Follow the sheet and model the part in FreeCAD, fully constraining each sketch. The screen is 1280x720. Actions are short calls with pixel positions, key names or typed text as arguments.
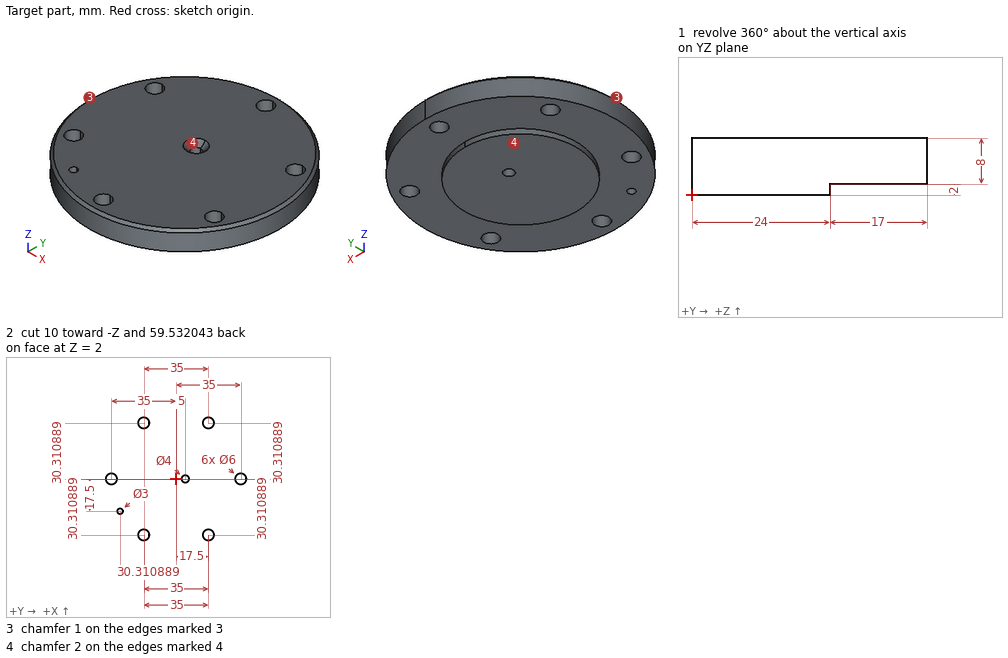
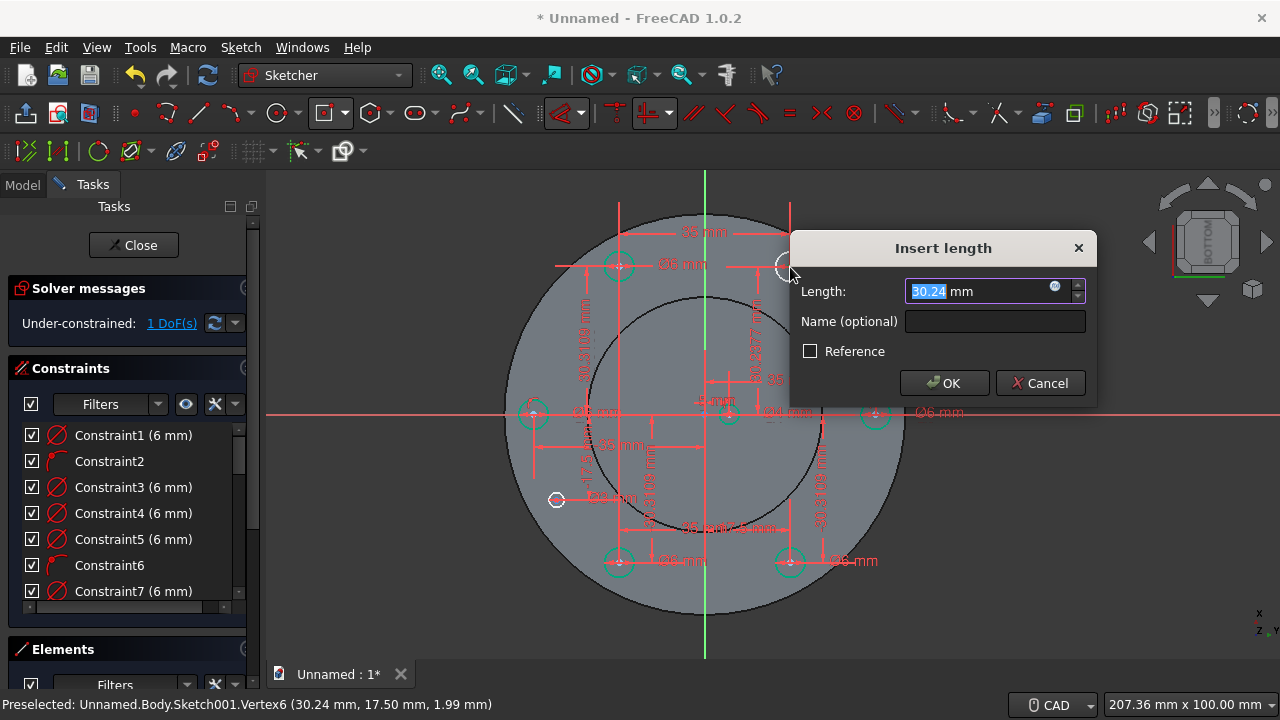
text(30.310889)
key(Return)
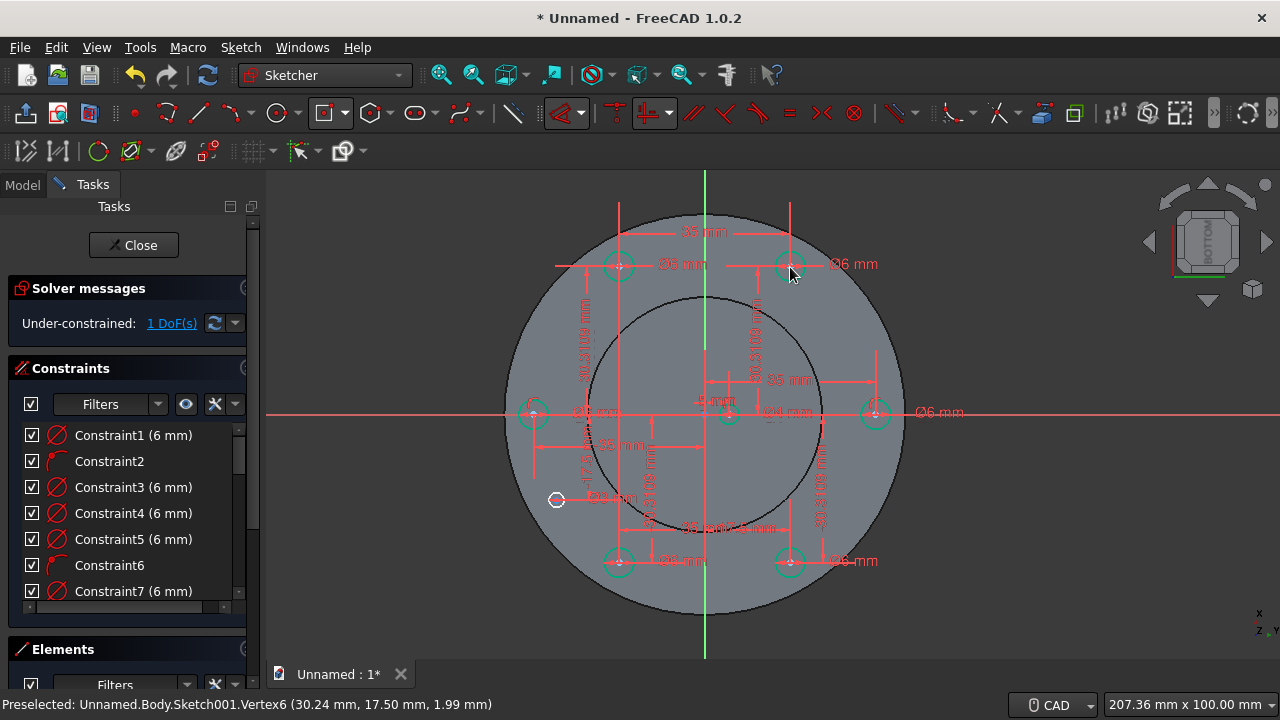
click(557, 500)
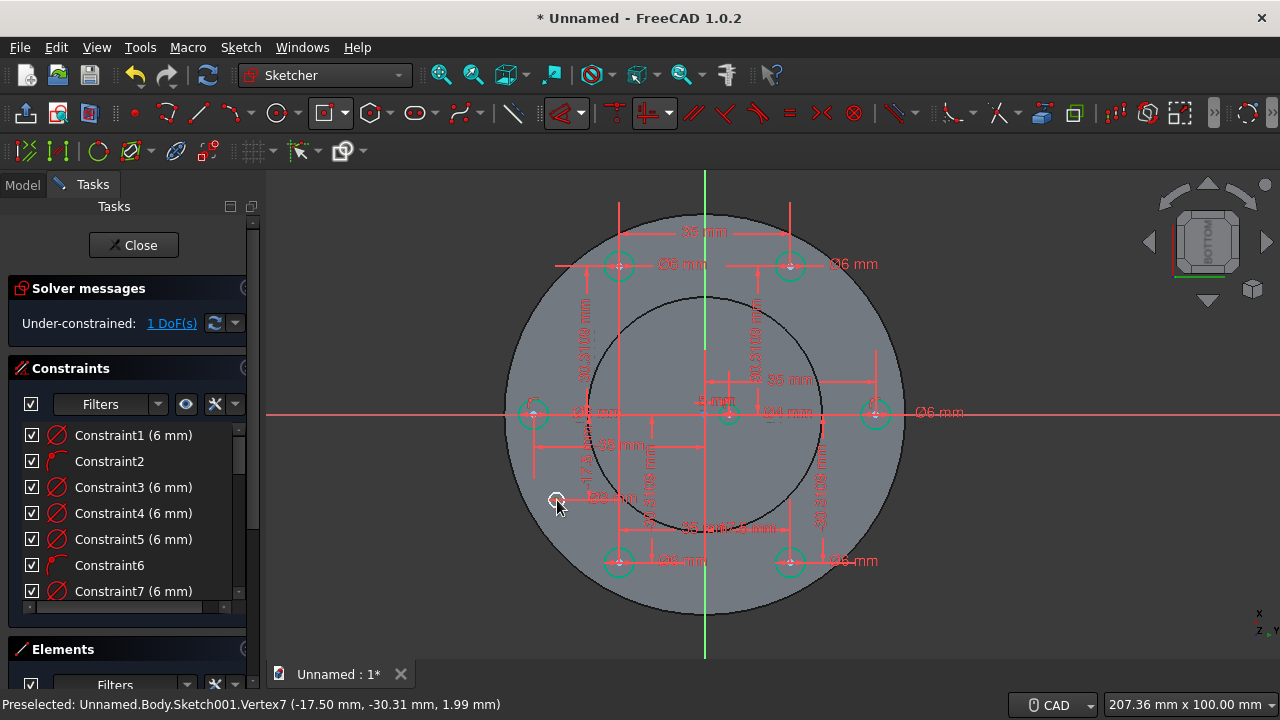
key(l)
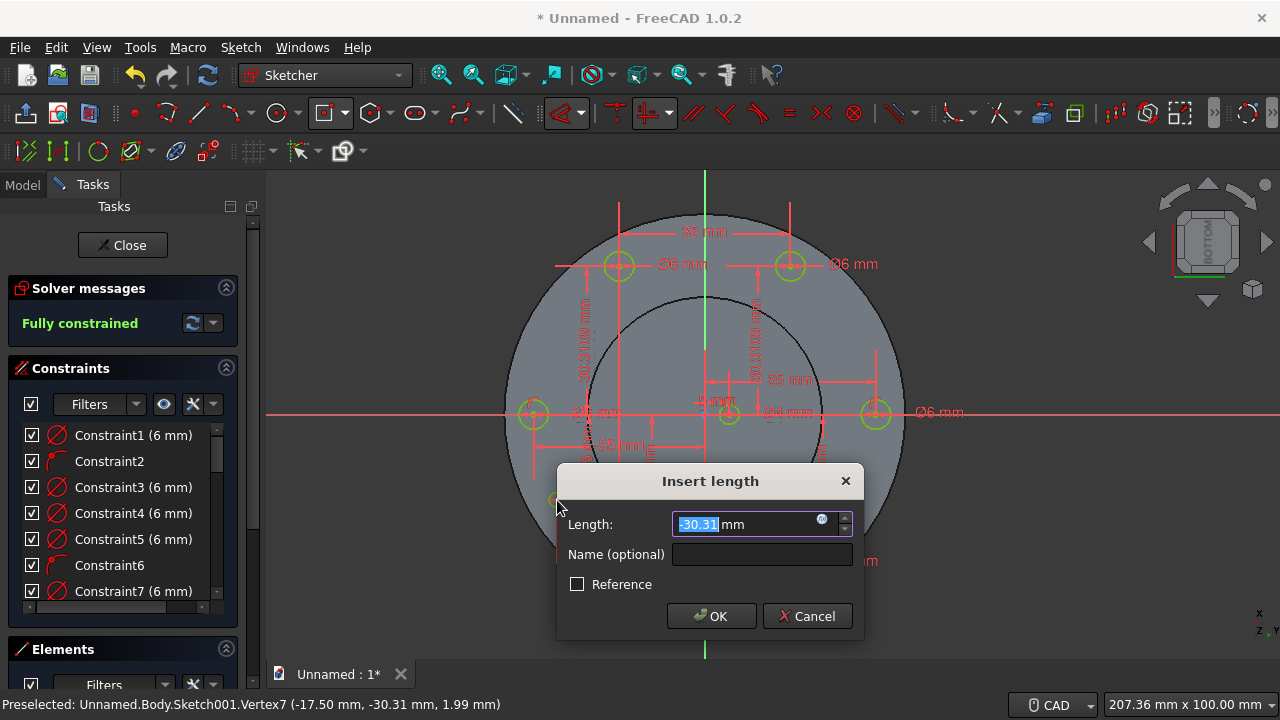
text(-30.310889)
key(Return)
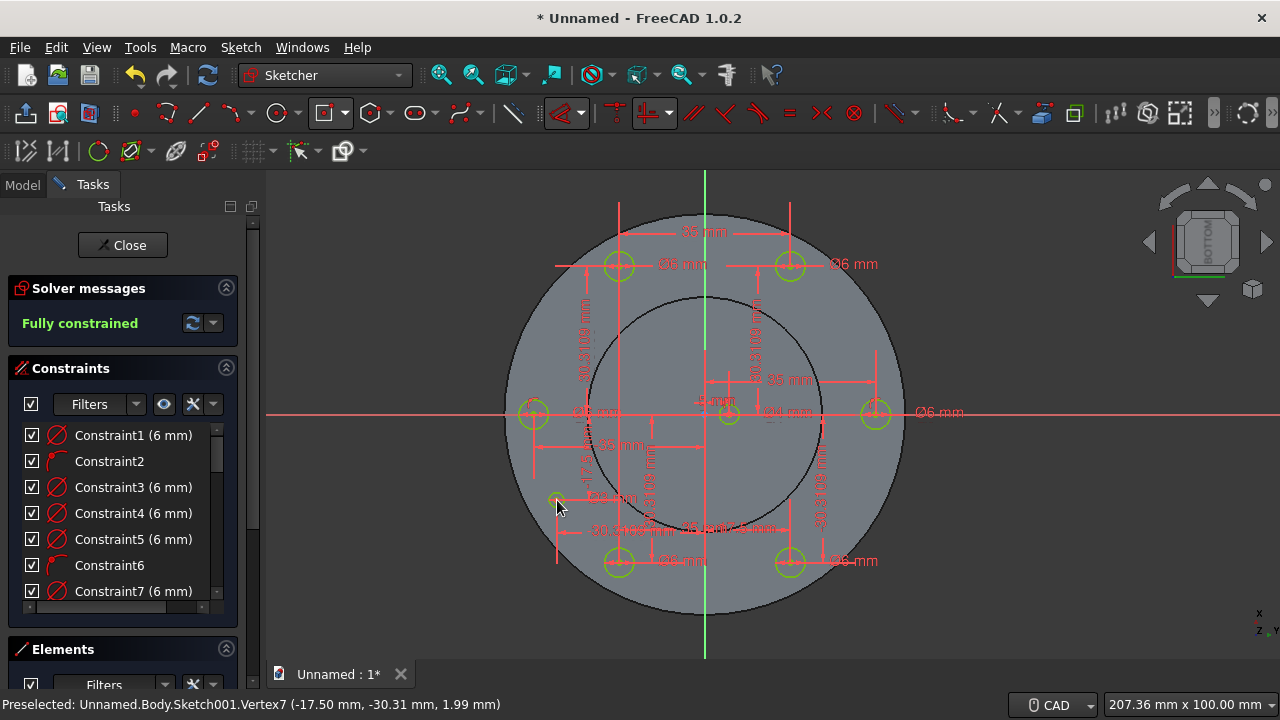
click(123, 245)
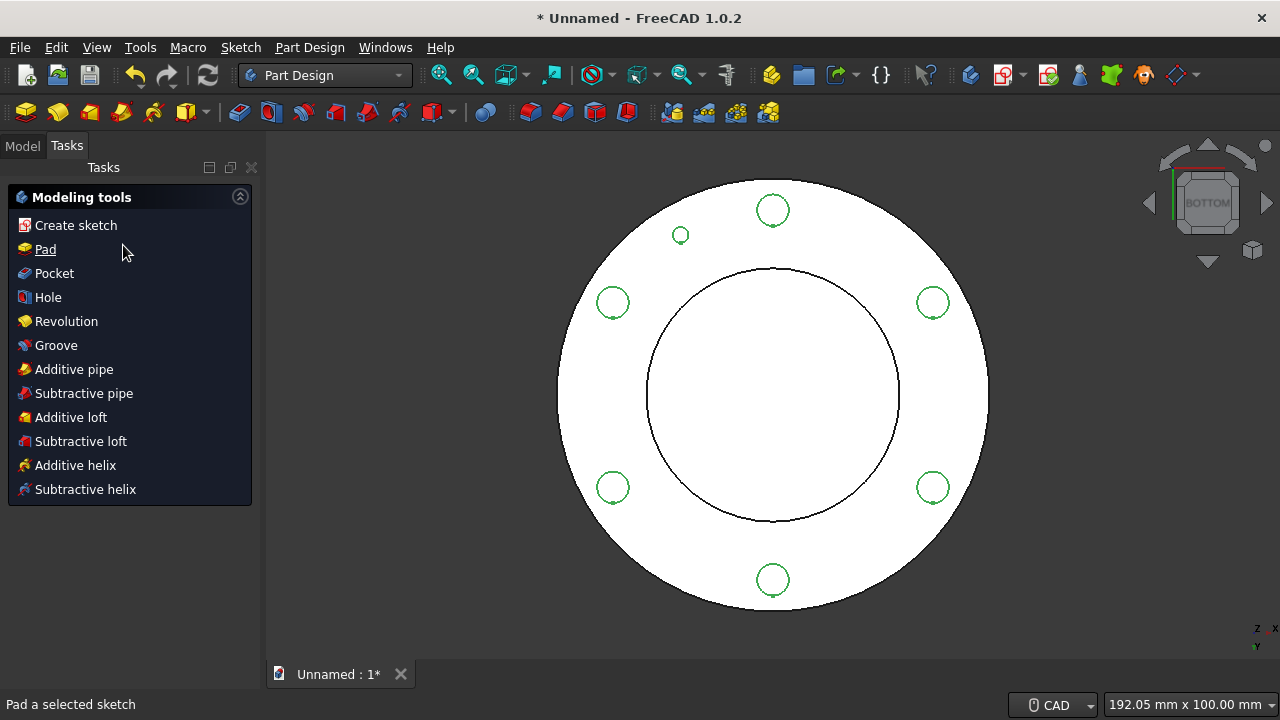
click(240, 112)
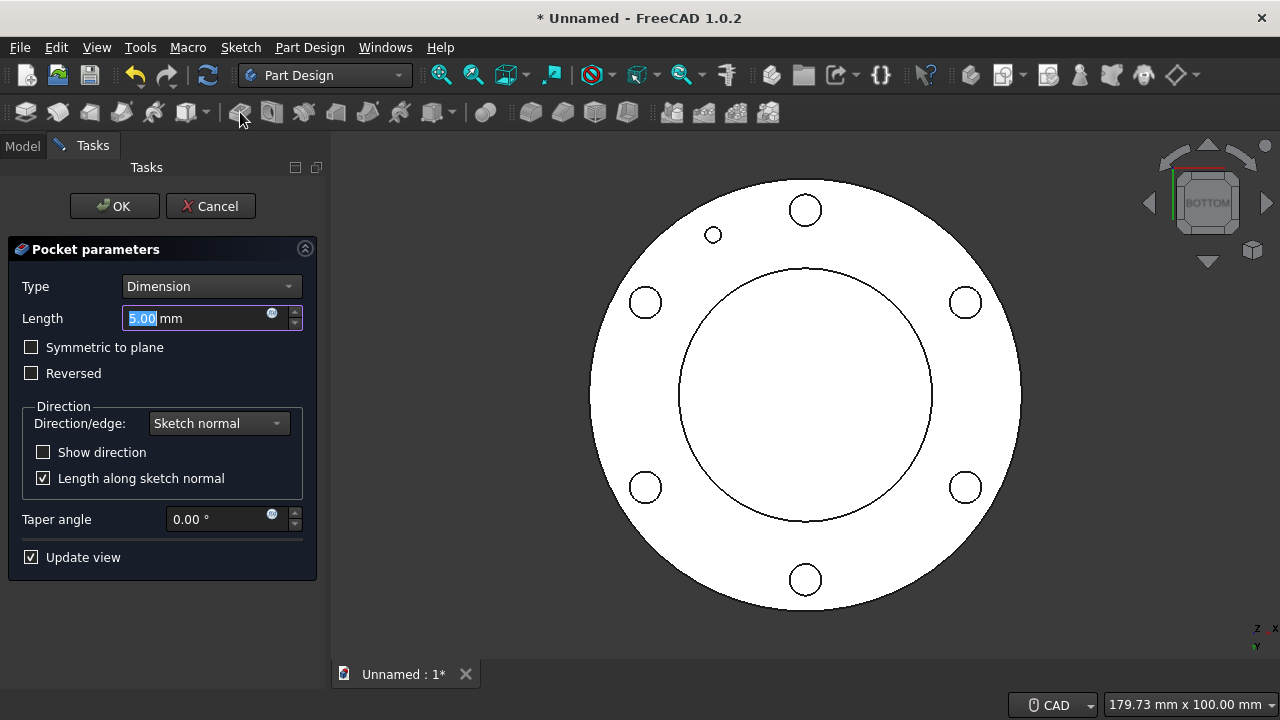
click(212, 286)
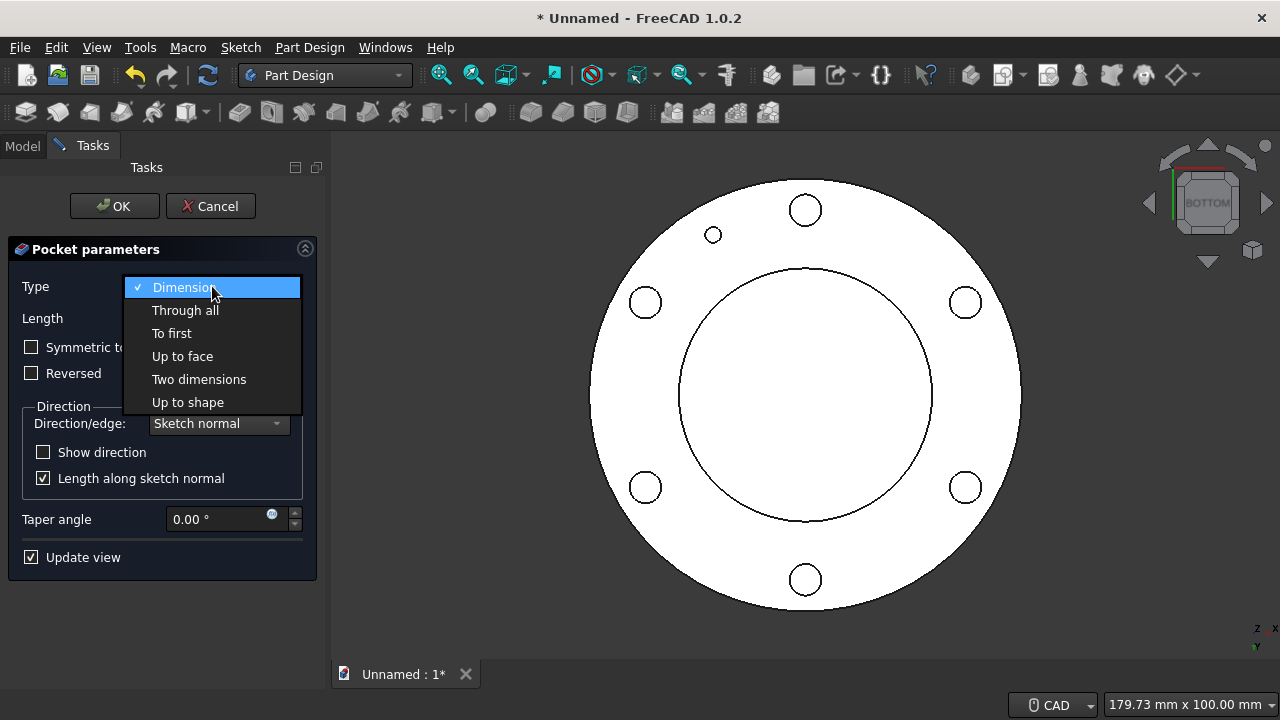
click(212, 380)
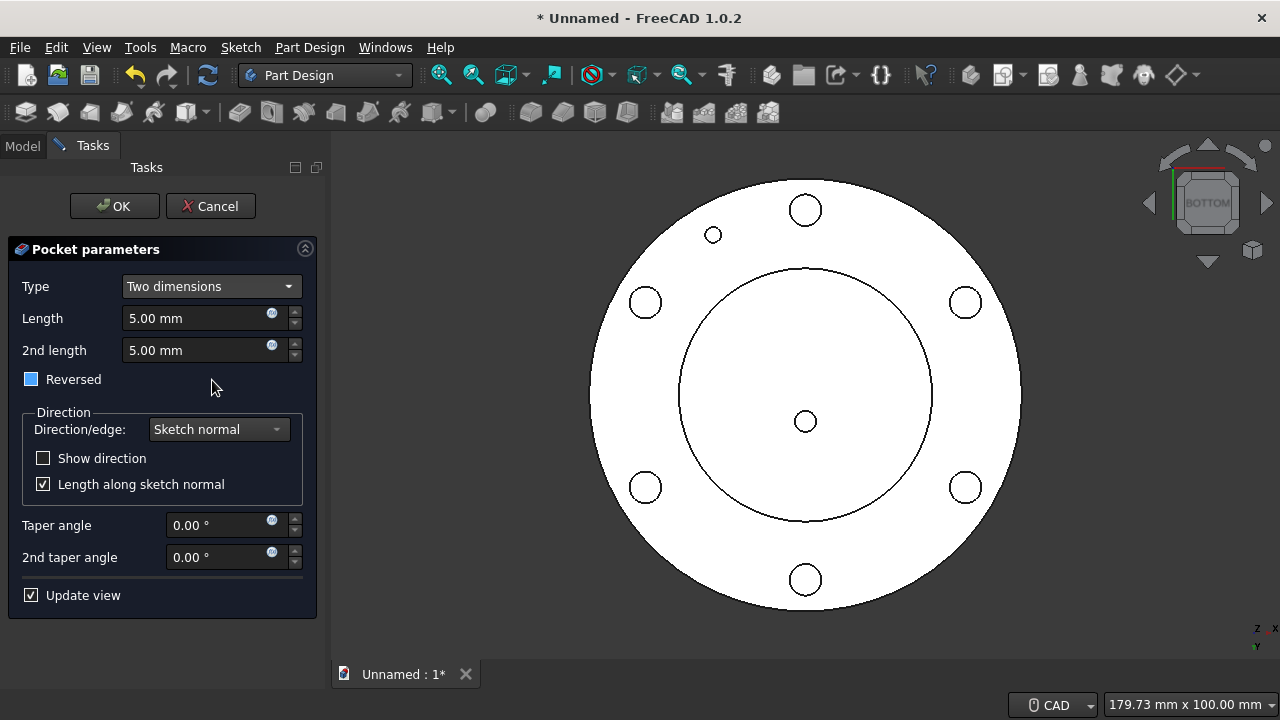
triple_click(204, 318)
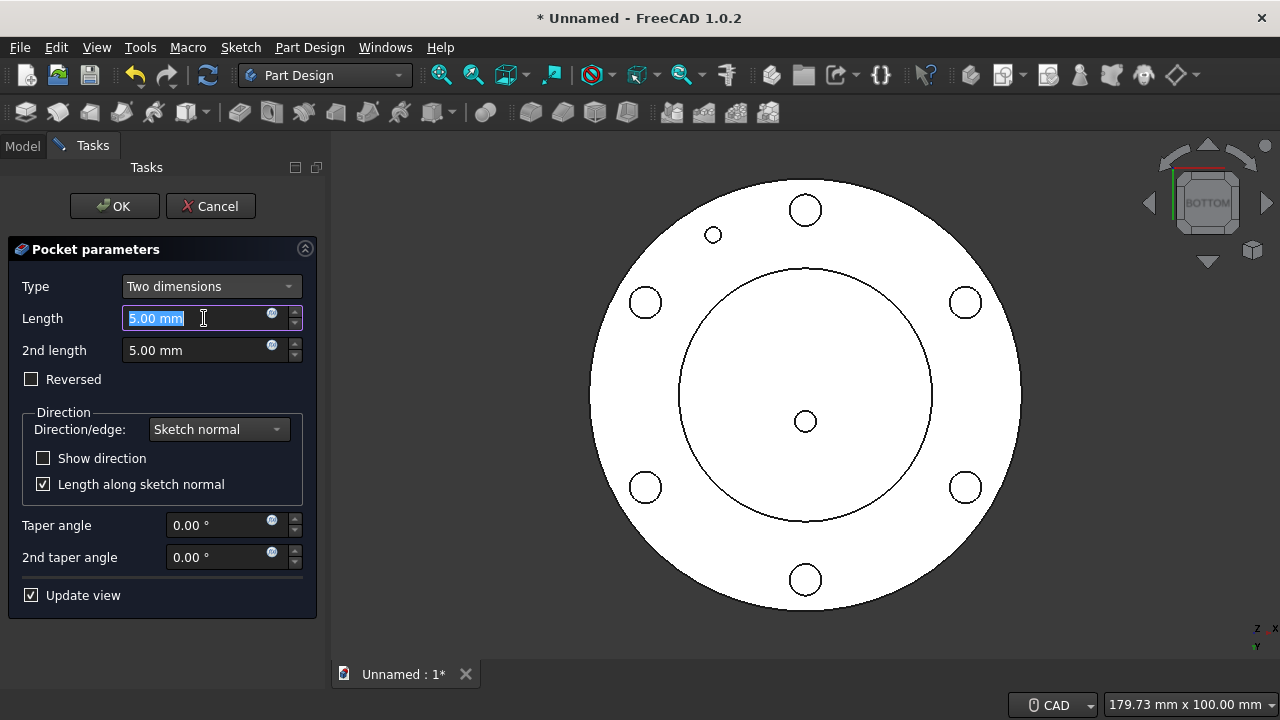
text(10)
key(Tab)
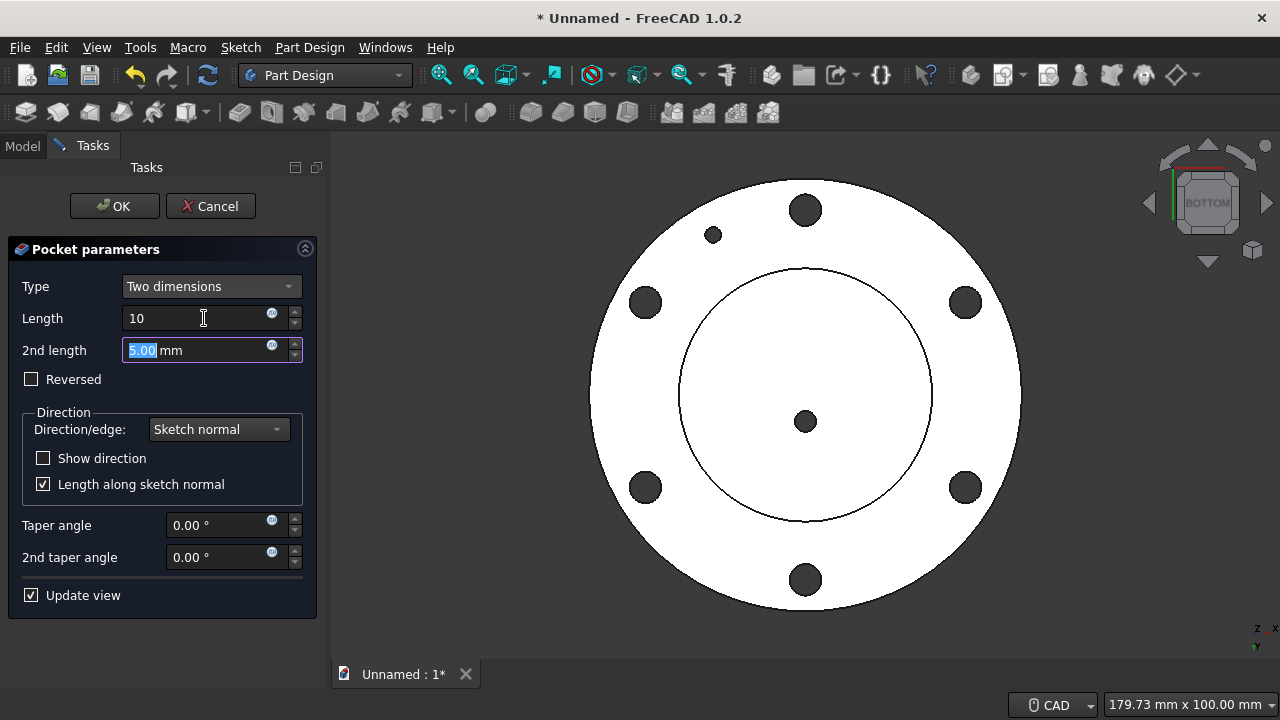
text(59.532043)
key(Tab)